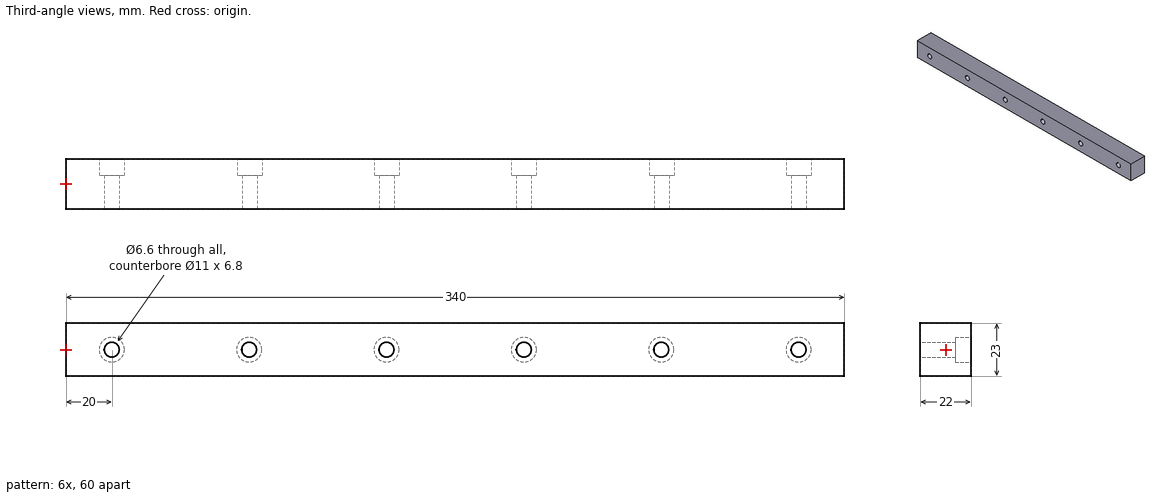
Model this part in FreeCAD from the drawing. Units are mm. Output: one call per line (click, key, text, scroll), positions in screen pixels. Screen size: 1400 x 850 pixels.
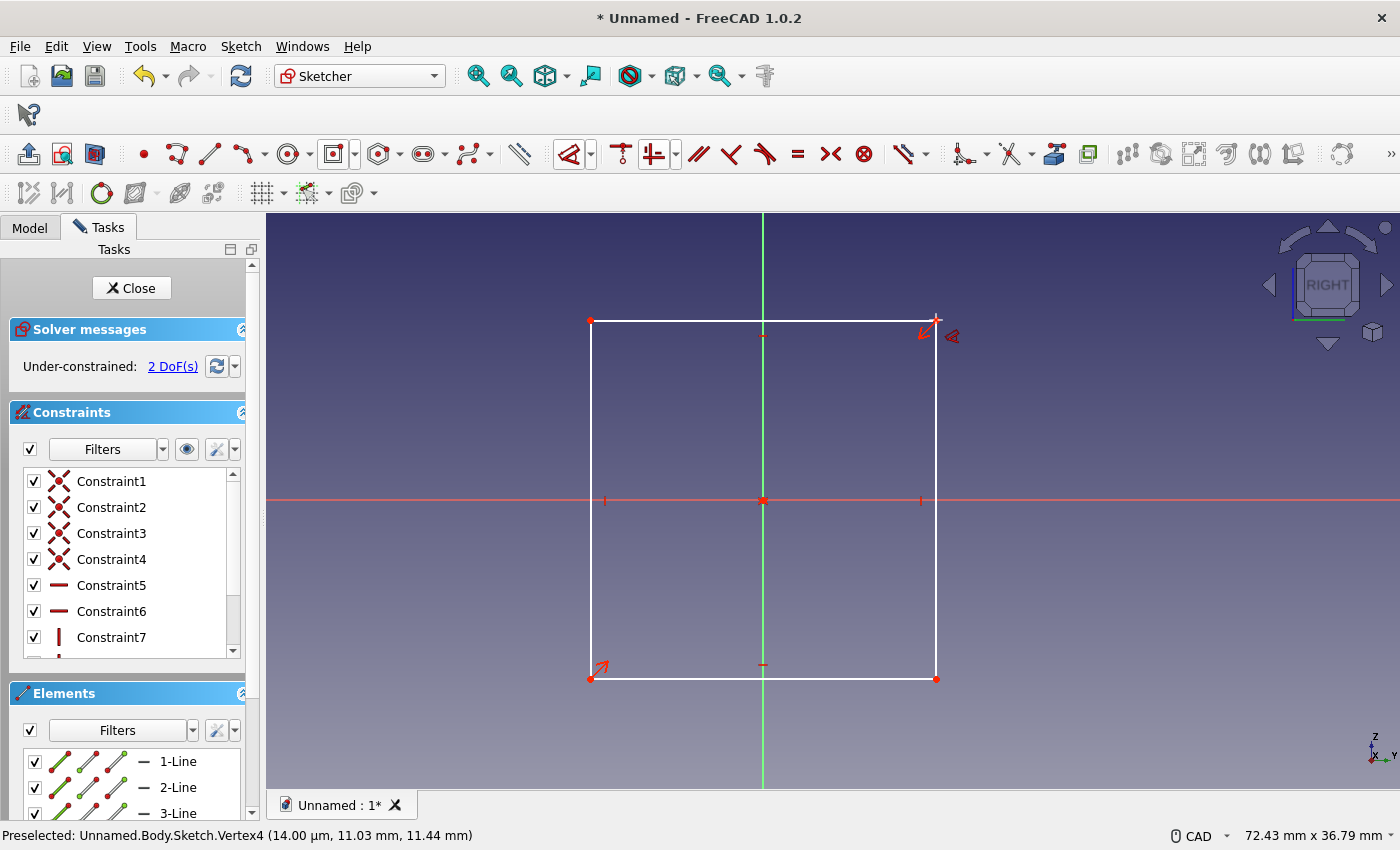
click(694, 679)
click(684, 713)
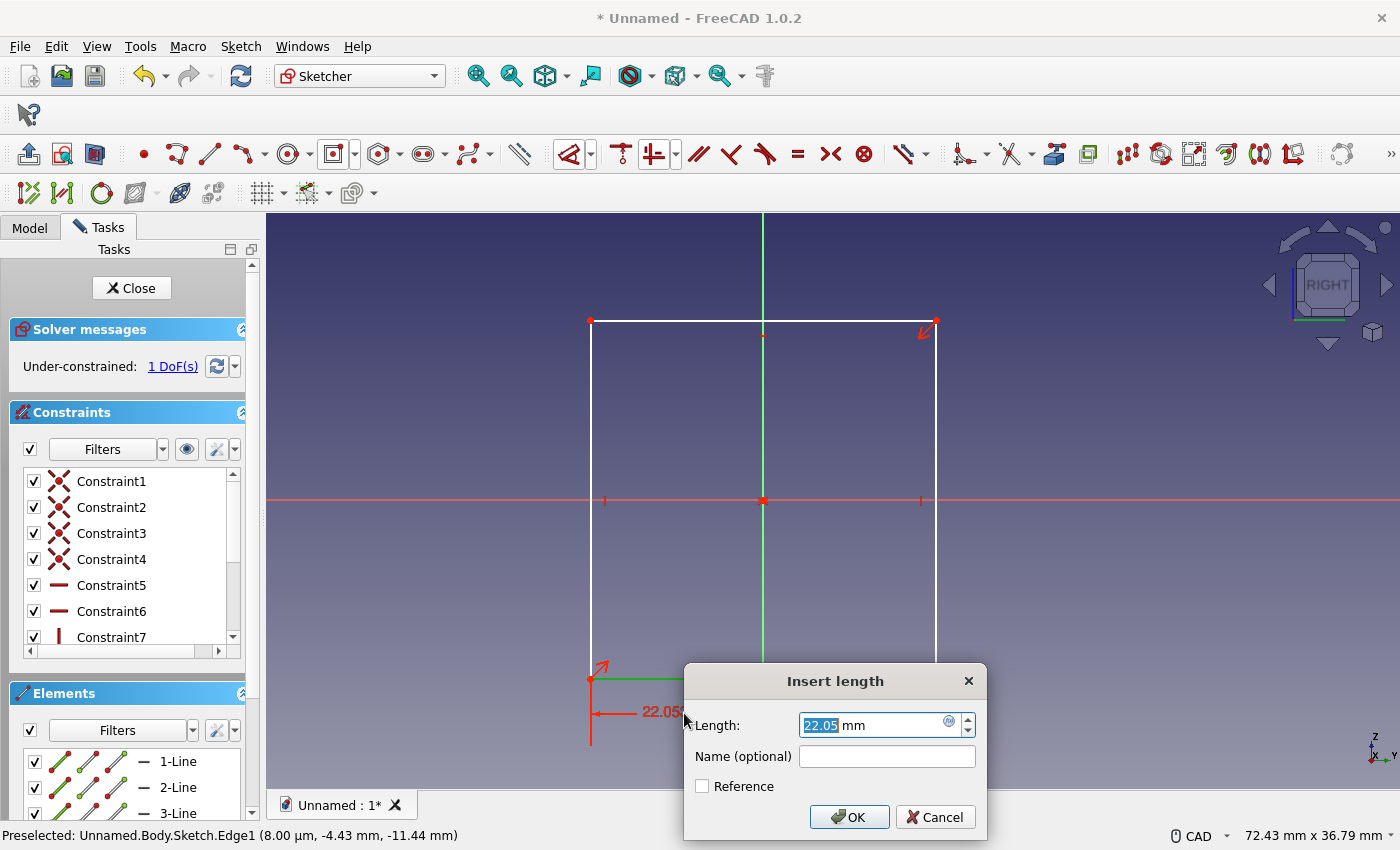
text(22)
key(Return)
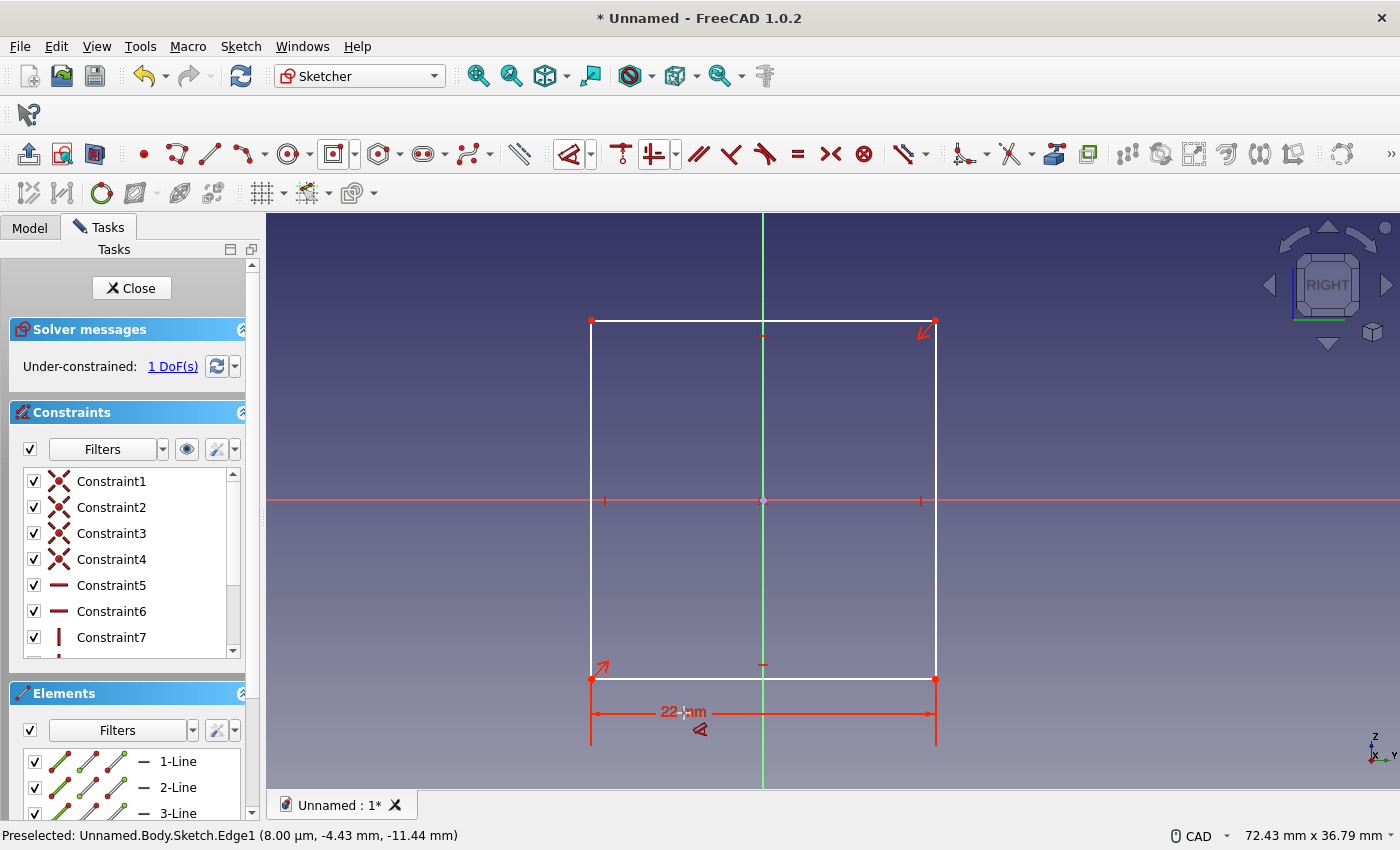
click(936, 572)
click(970, 418)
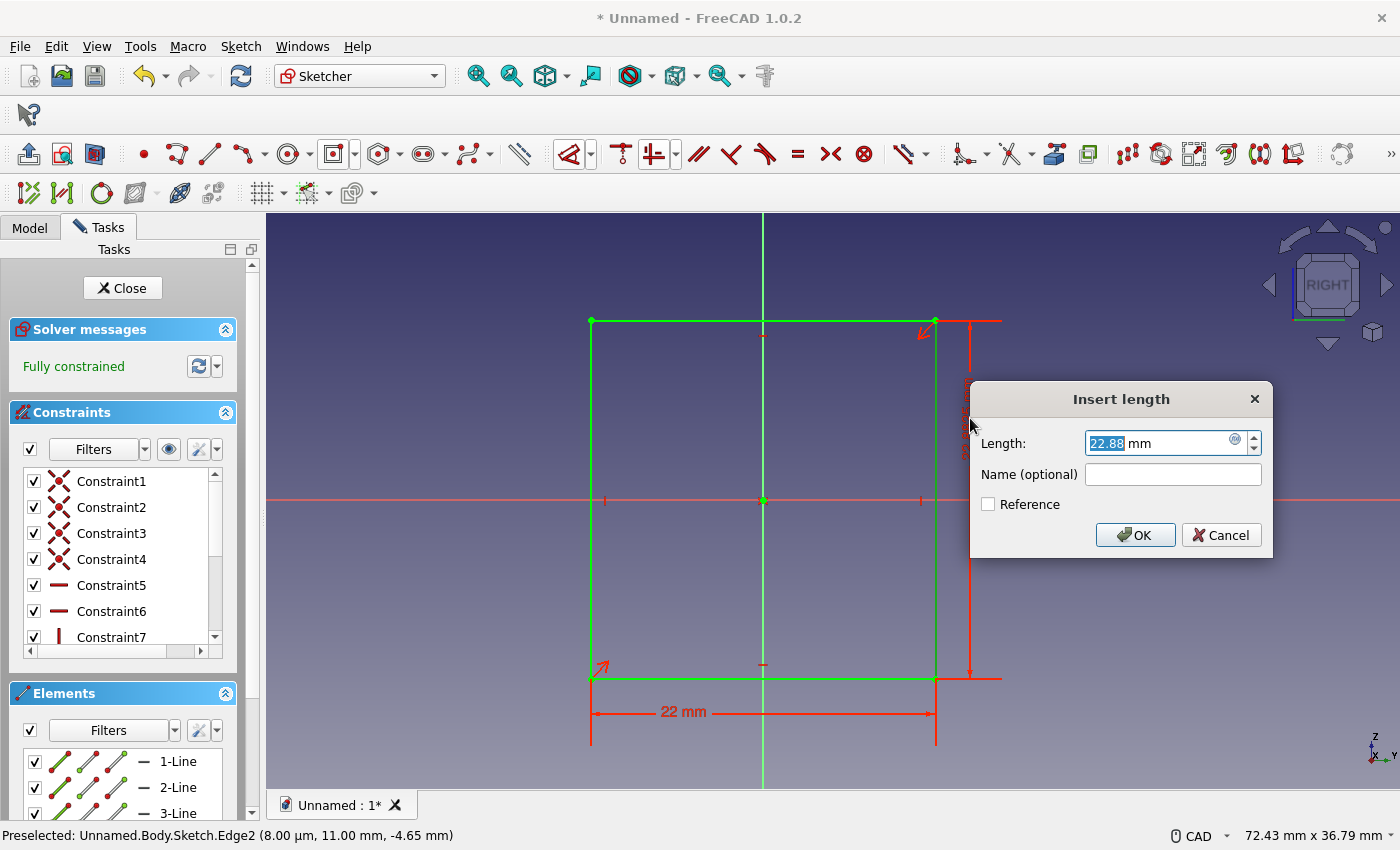
text(23)
key(Return)
key(Escape)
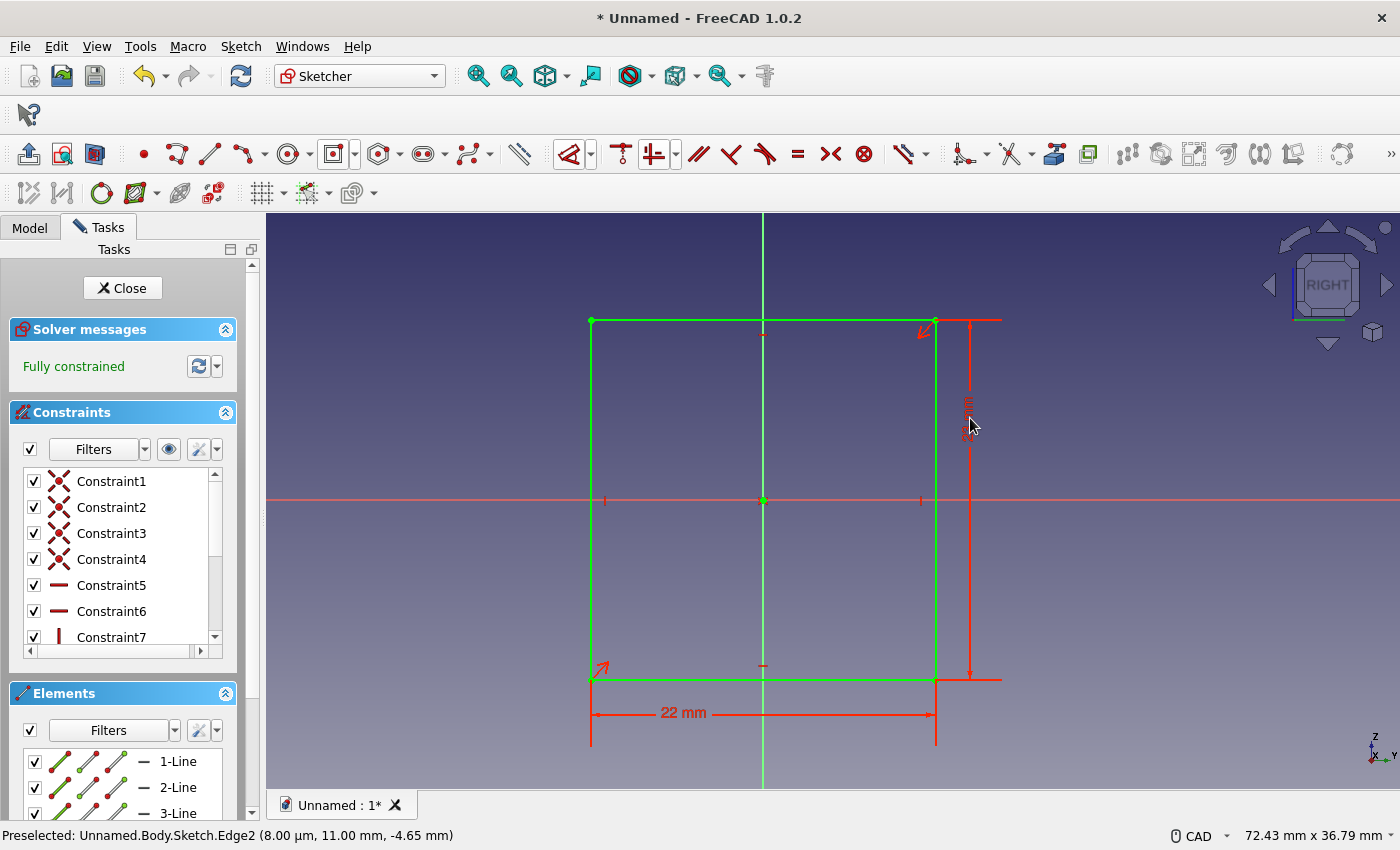
click(123, 288)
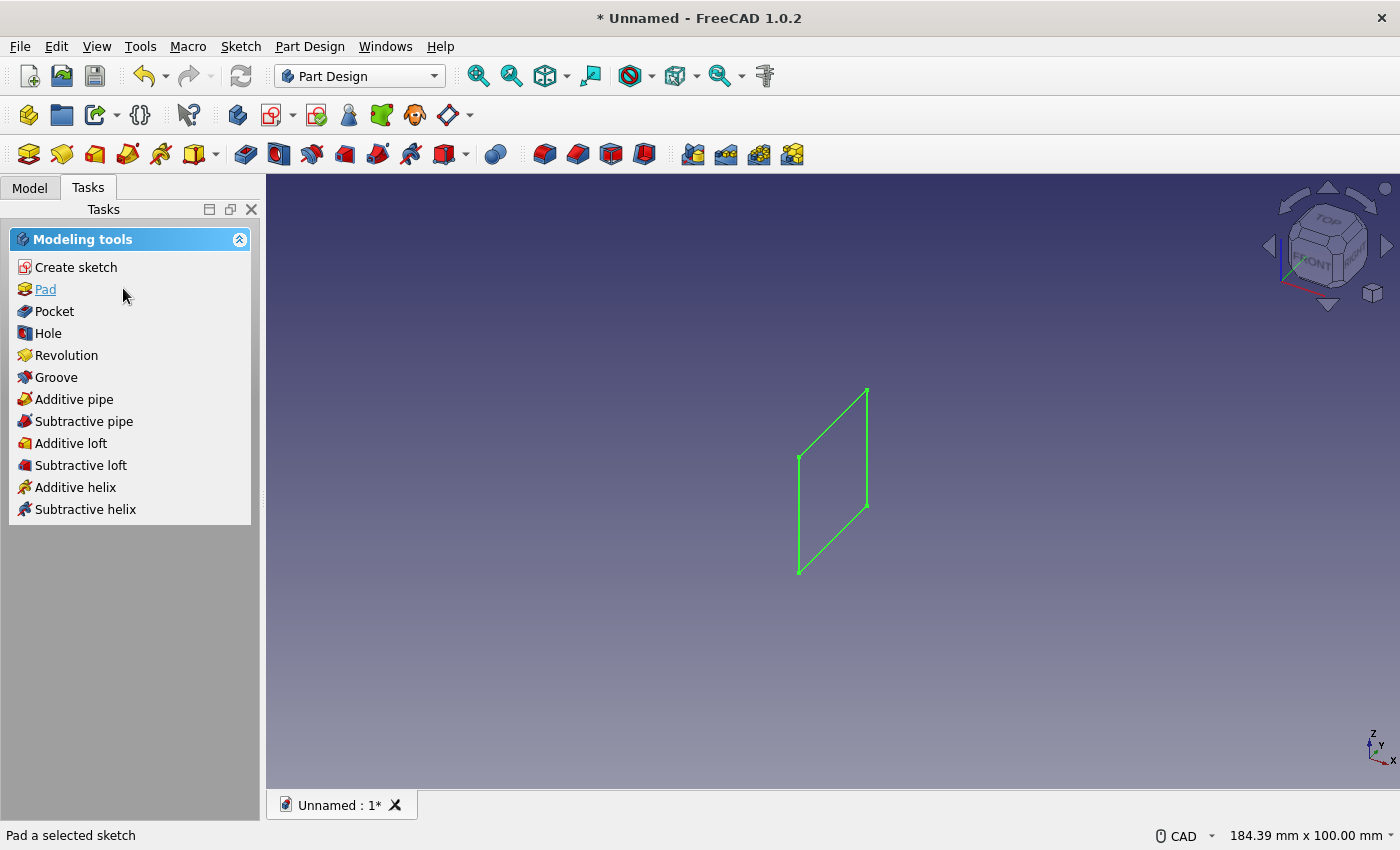
click(29, 154)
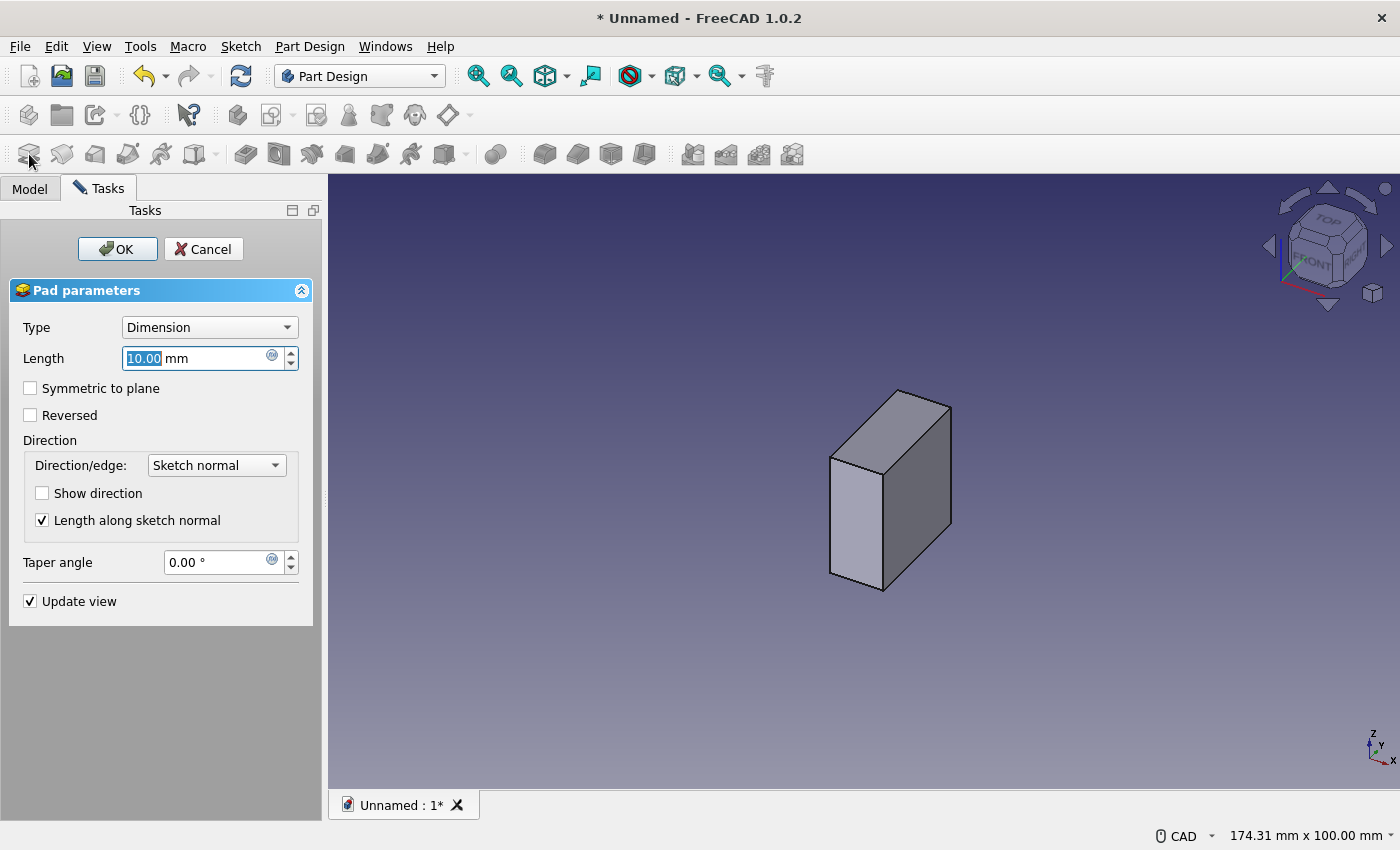
text(340)
key(Tab)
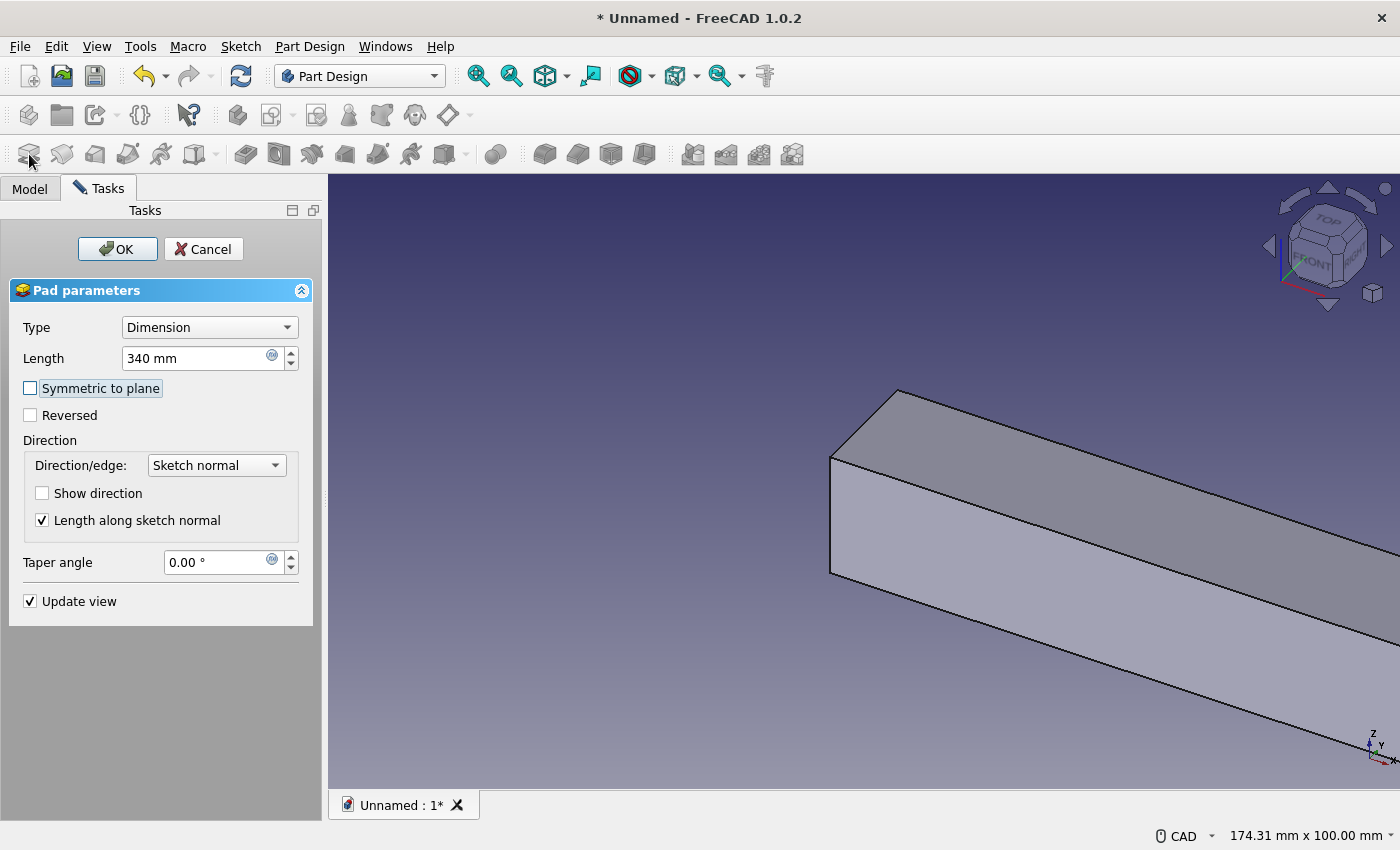
click(118, 249)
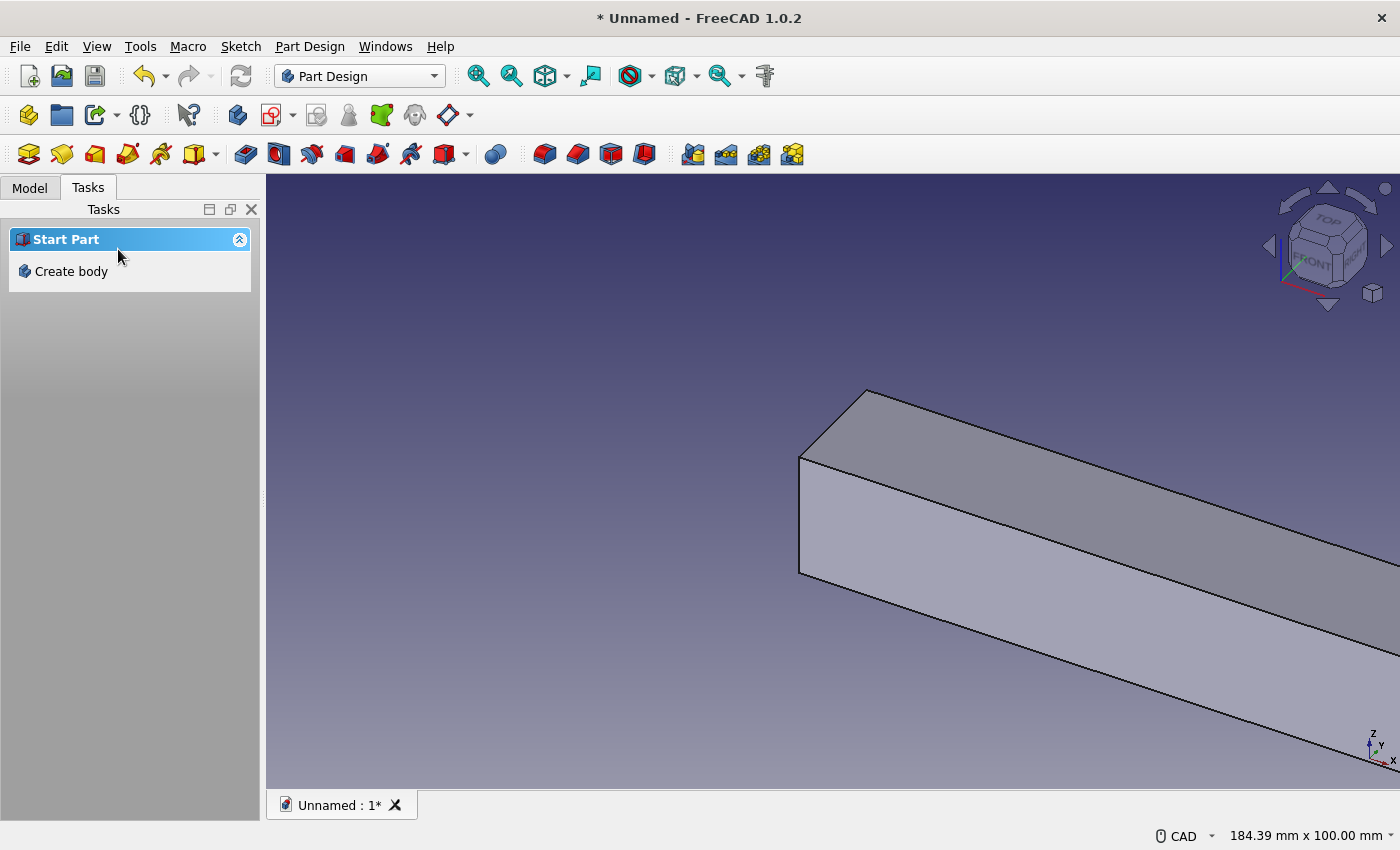
click(479, 76)